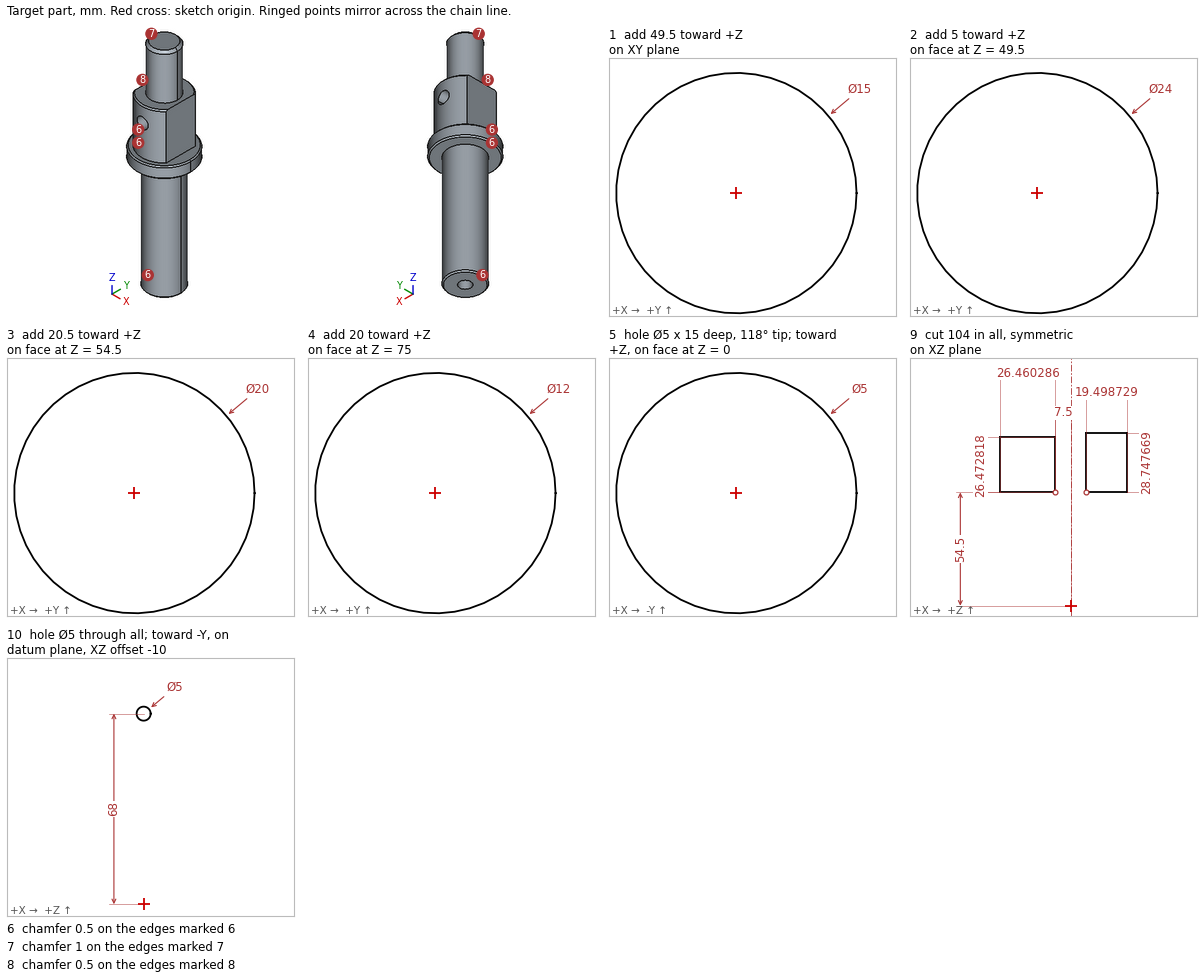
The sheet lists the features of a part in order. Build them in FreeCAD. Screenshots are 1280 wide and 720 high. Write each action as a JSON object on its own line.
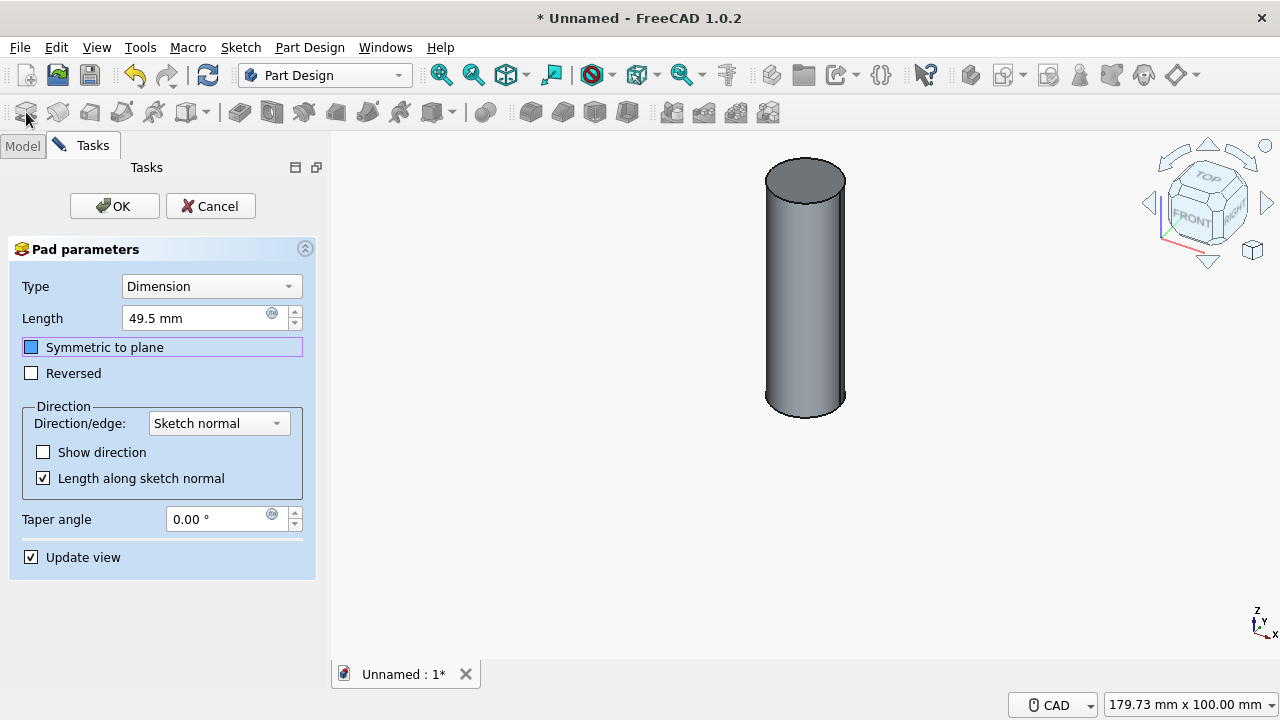
{"action": "left_click", "coordinate": [115, 206]}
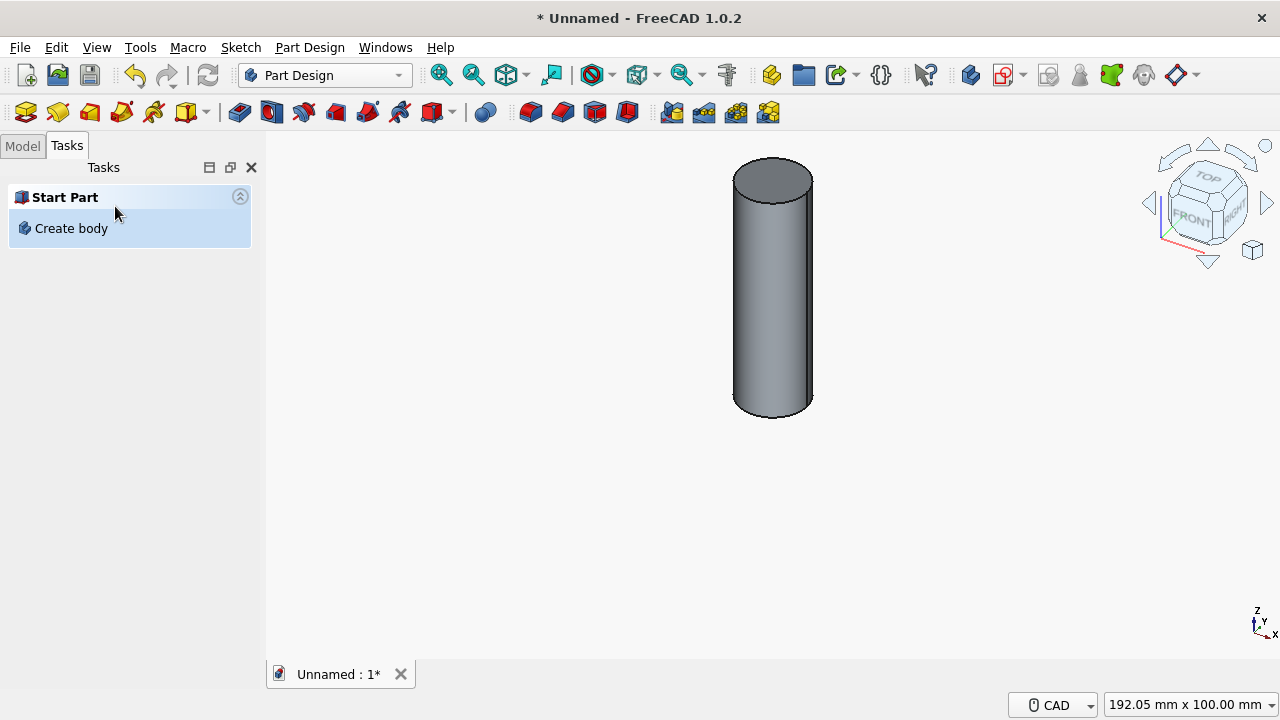
{"action": "left_click", "coordinate": [773, 180]}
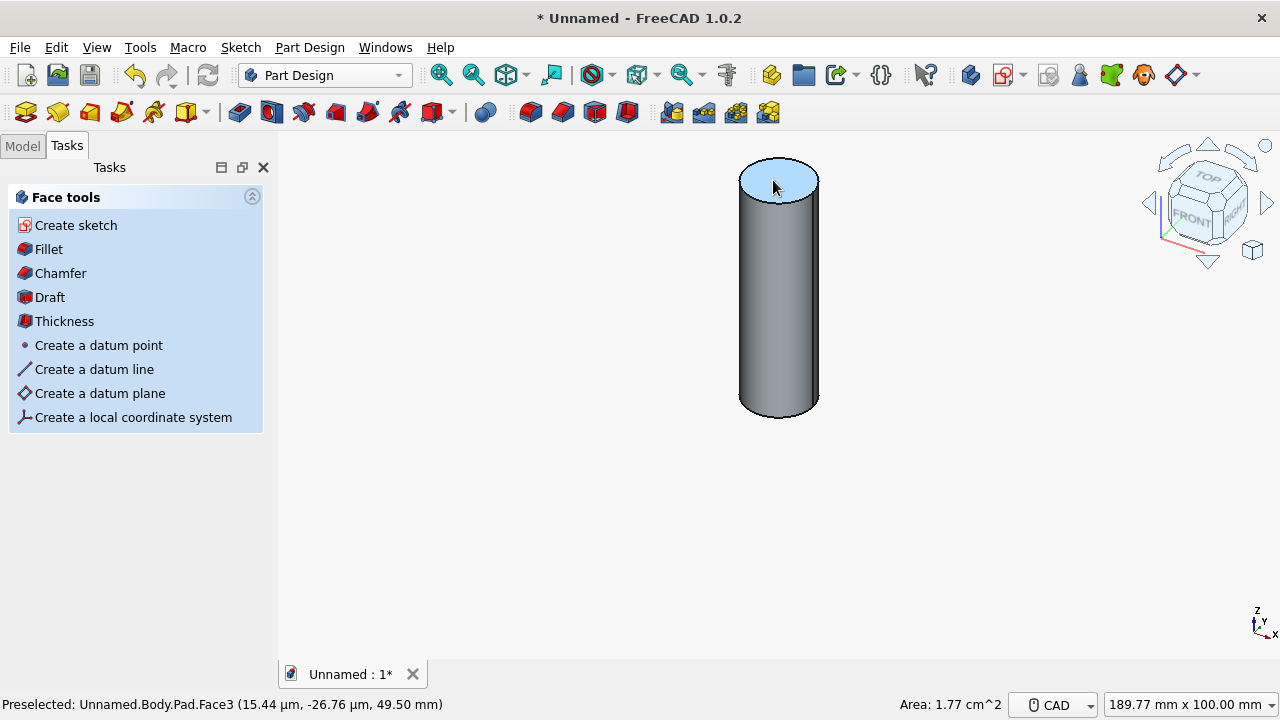
{"action": "left_click", "coordinate": [1004, 76]}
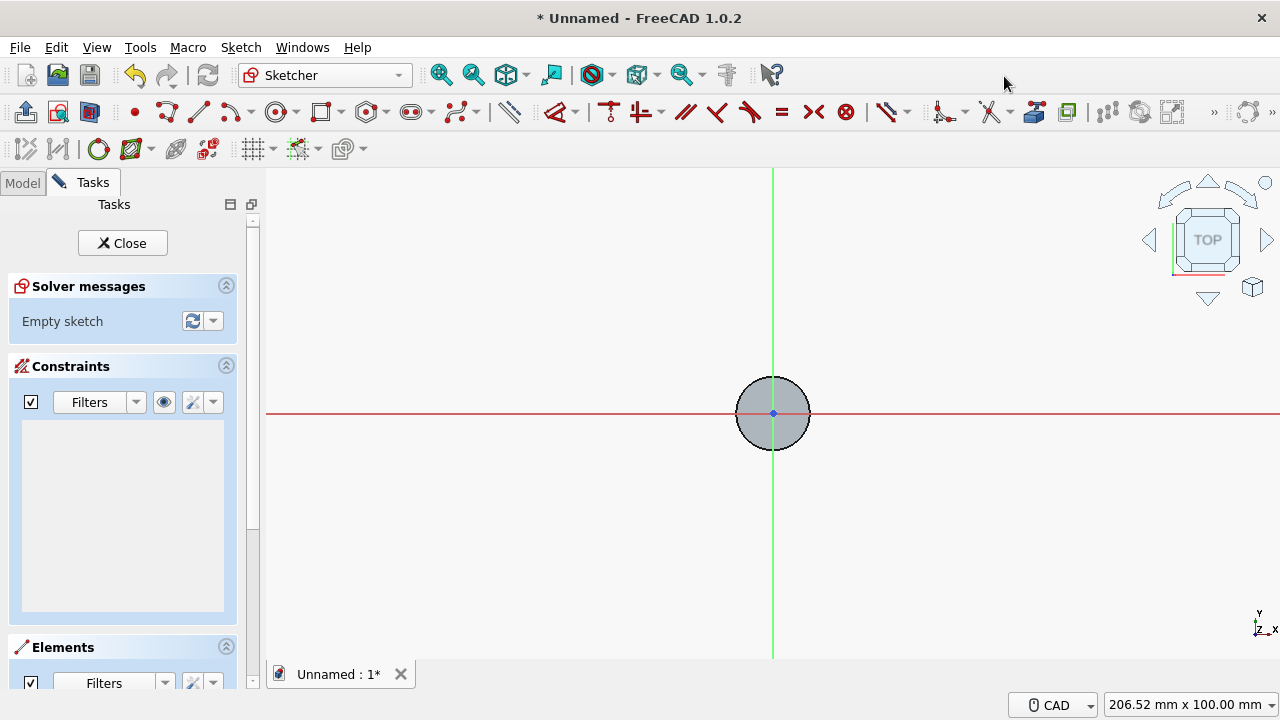
{"action": "scroll", "coordinate": [813, 414], "scroll_direction": "up", "scroll_amount": 5}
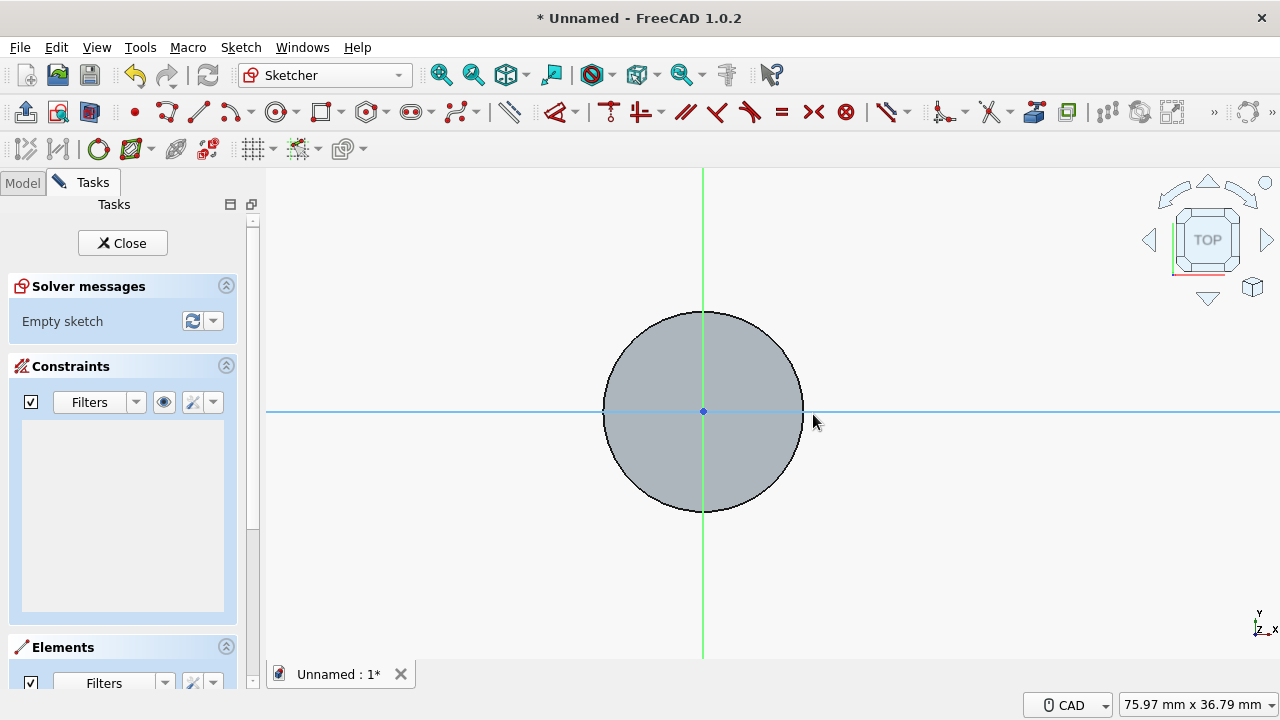
{"action": "key", "text": "g c"}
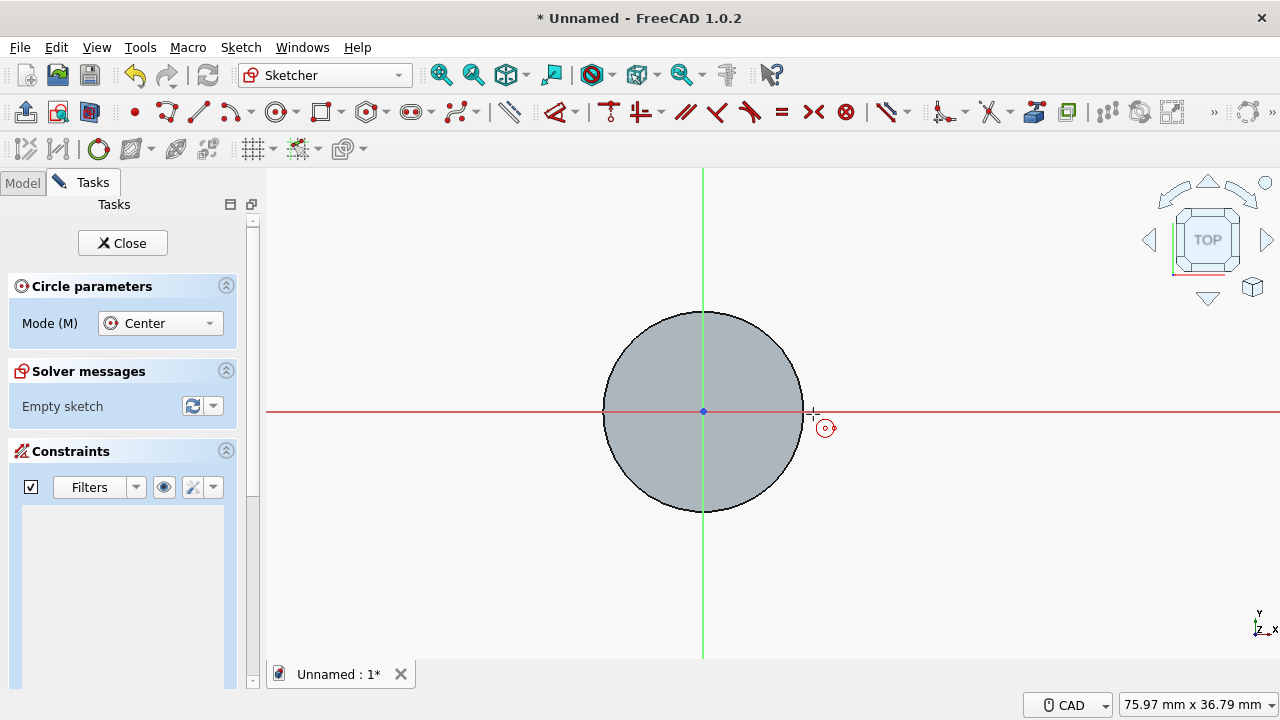
{"action": "left_click", "coordinate": [703, 412]}
{"action": "mouse_move", "coordinate": [817, 299]}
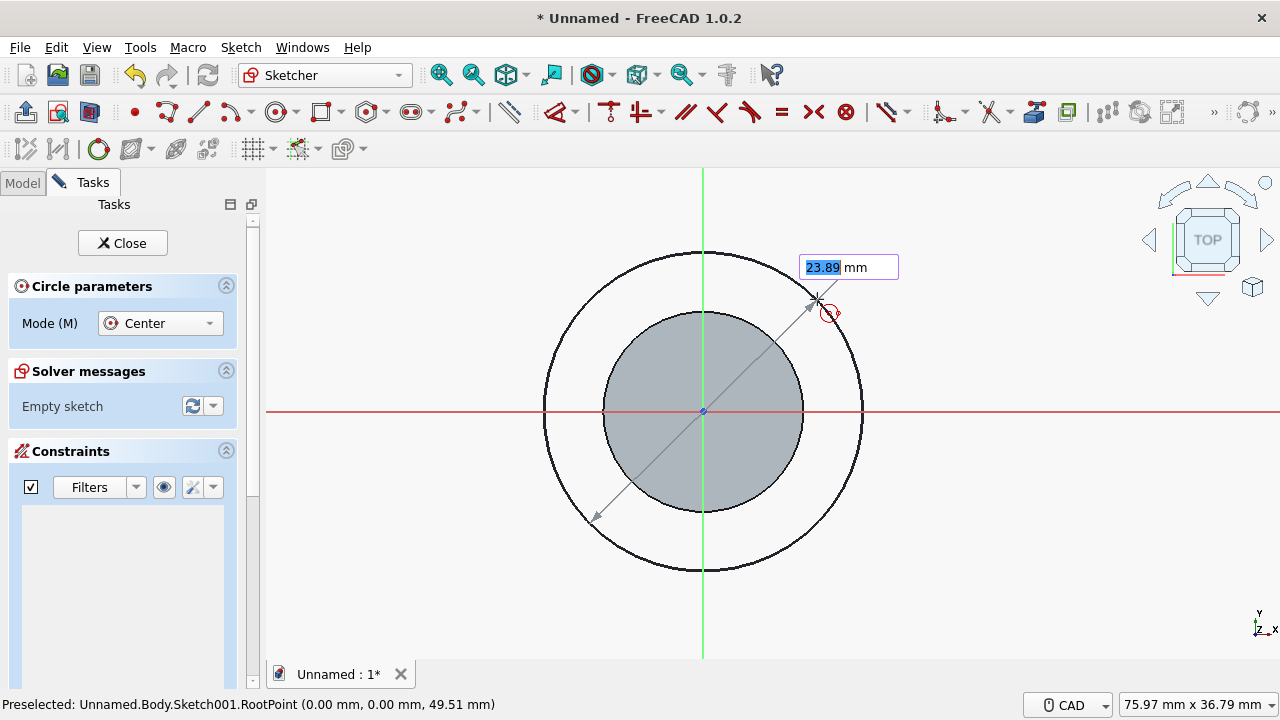
{"action": "type", "text": "24"}
{"action": "key", "text": "Return"}
{"action": "key", "text": "Escape"}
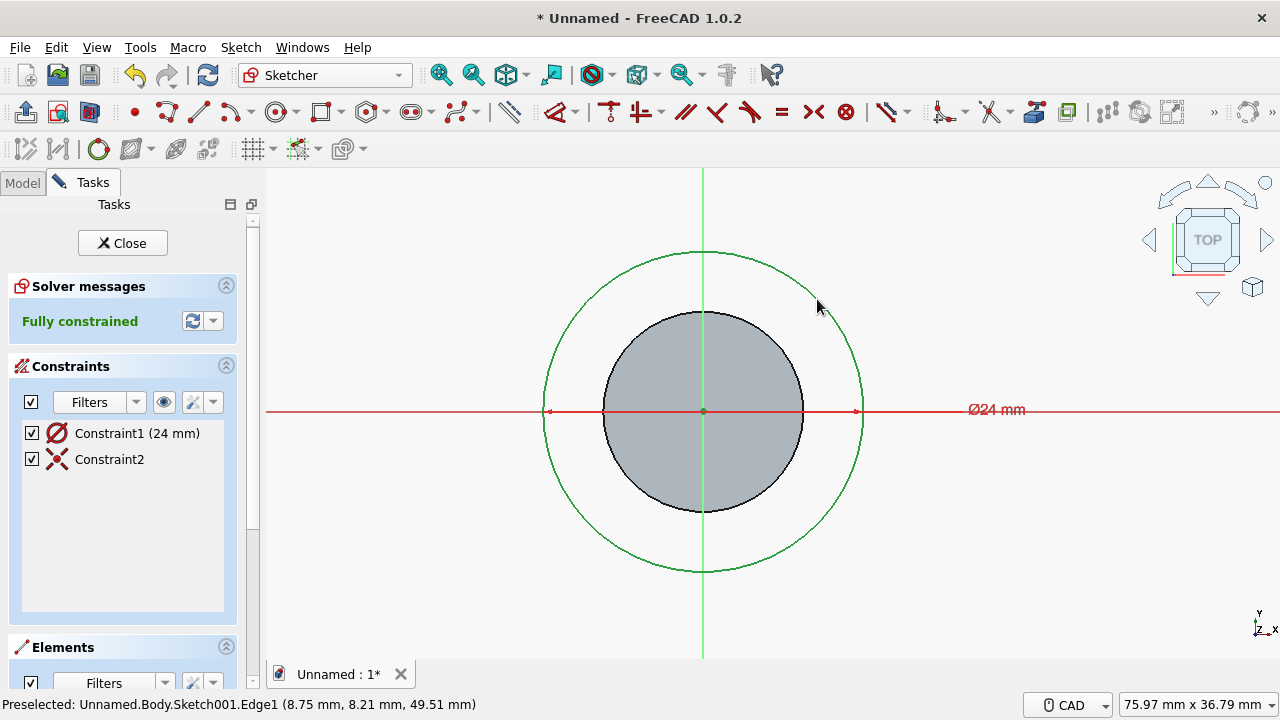
{"action": "left_click", "coordinate": [123, 243]}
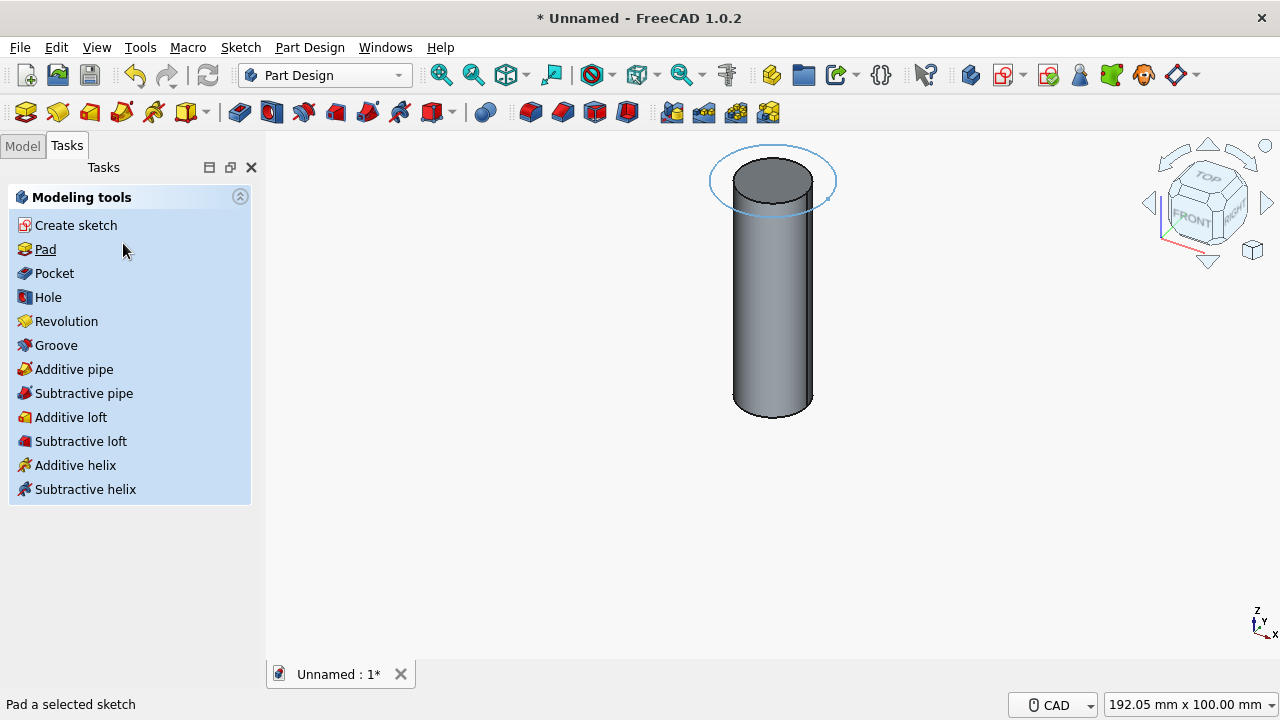
{"action": "left_click", "coordinate": [26, 112]}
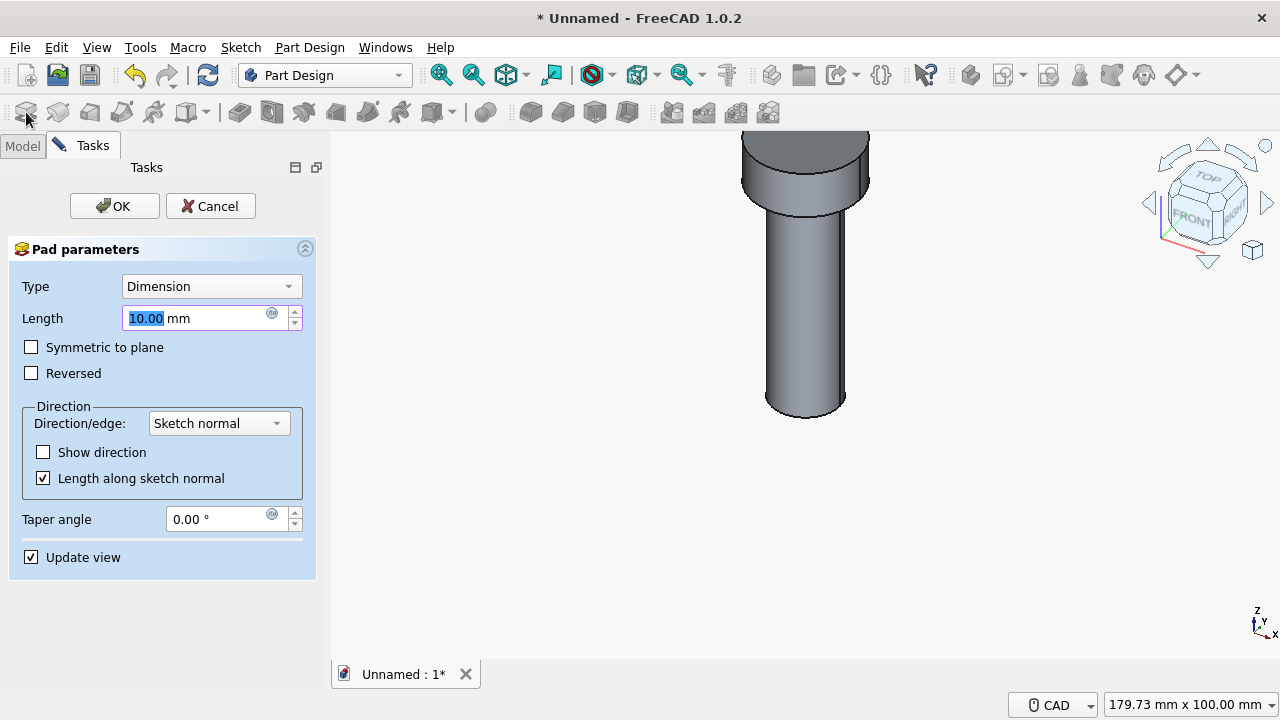
{"action": "type", "text": "5"}
{"action": "key", "text": "Tab"}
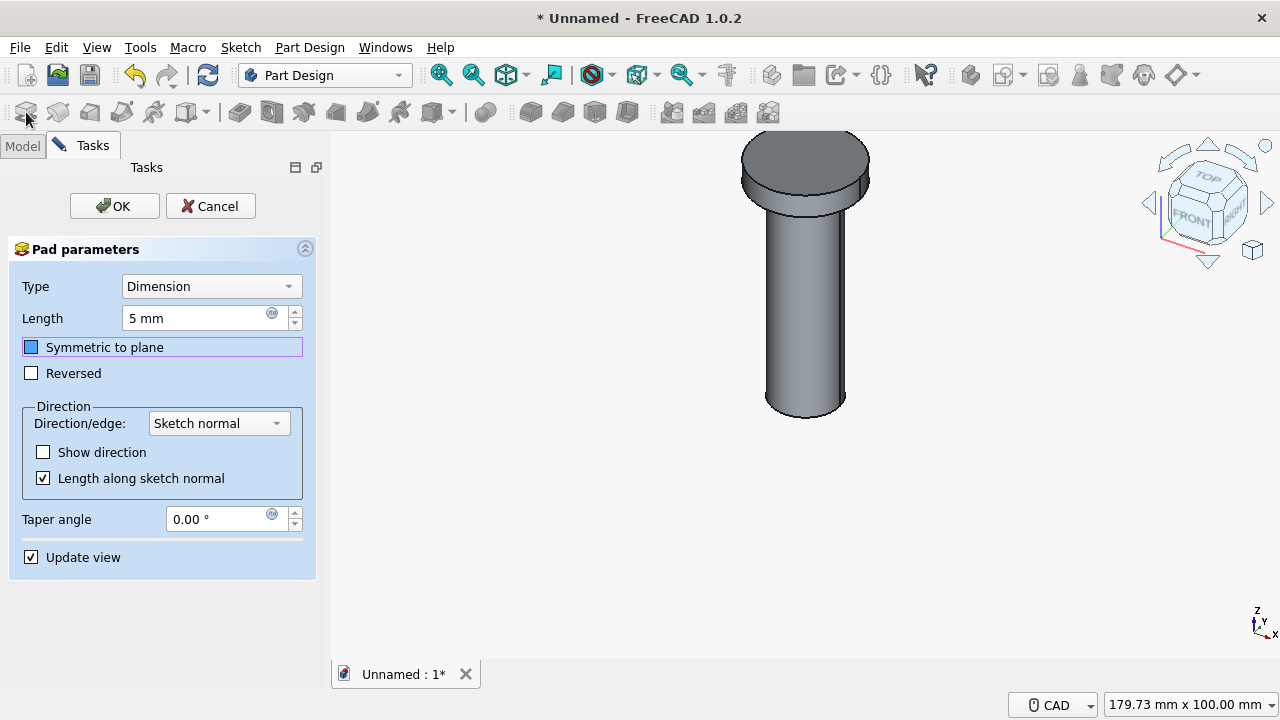
{"action": "left_click", "coordinate": [115, 206]}